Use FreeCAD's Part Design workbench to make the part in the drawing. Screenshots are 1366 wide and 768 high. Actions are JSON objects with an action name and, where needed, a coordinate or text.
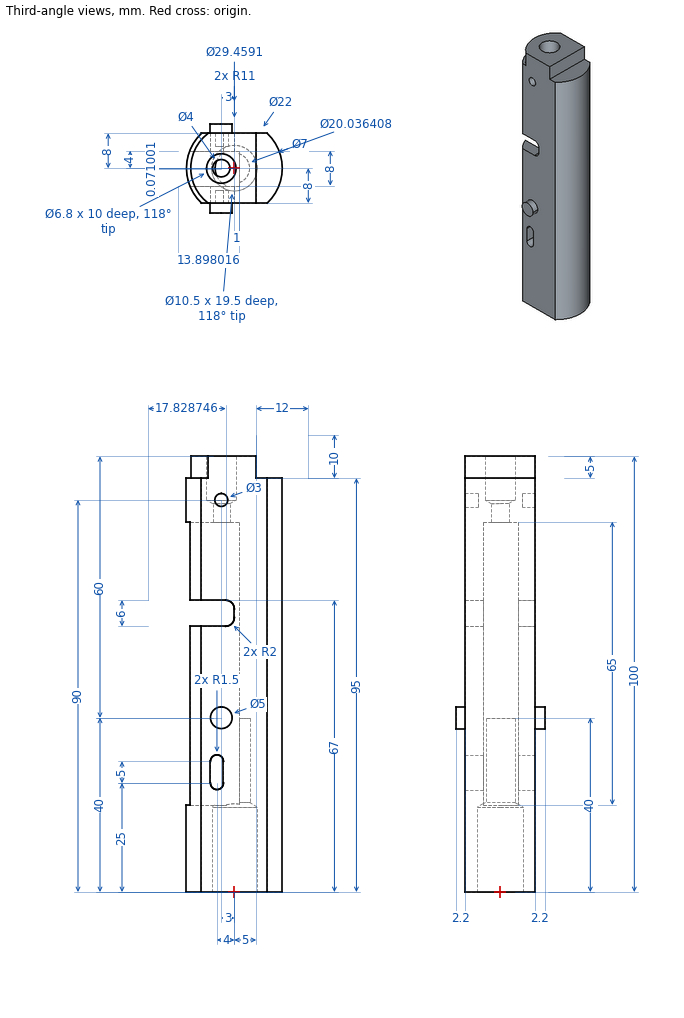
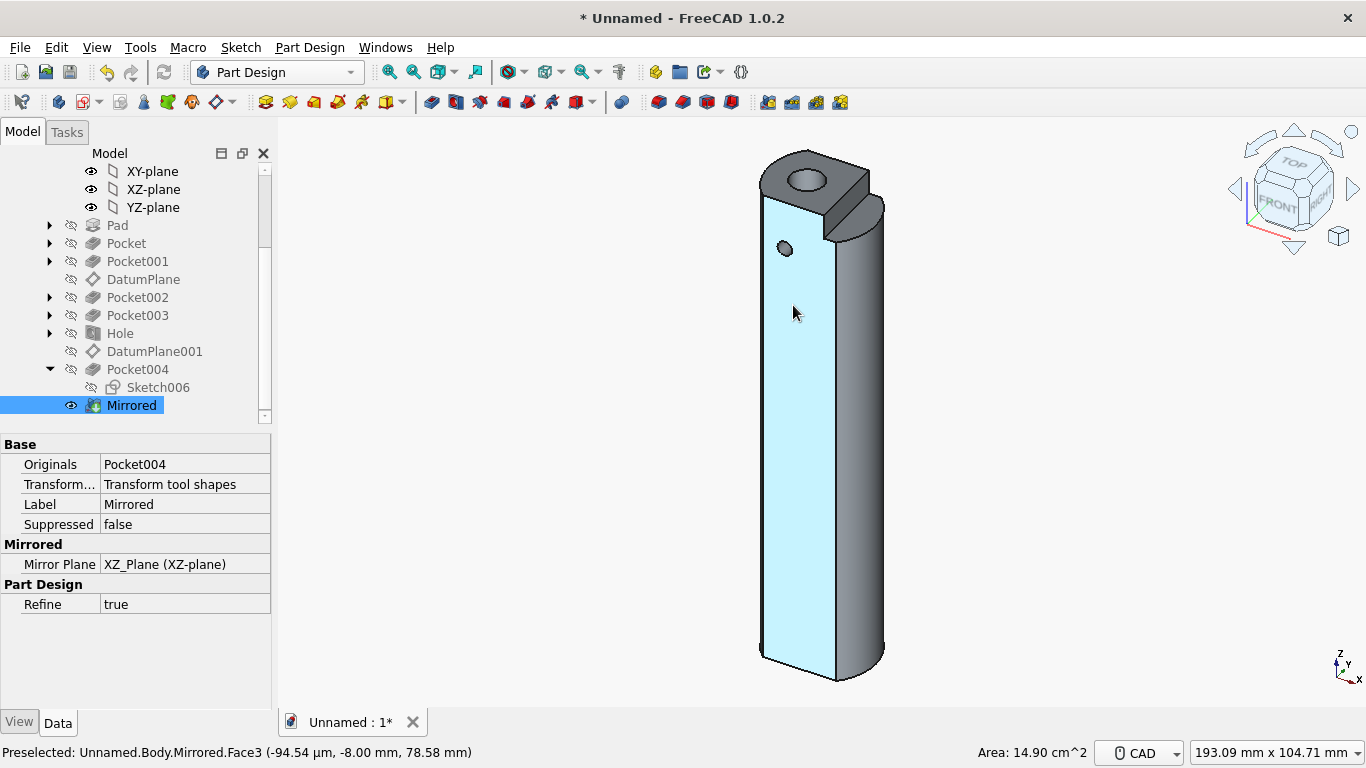
{"action": "left_click", "coordinate": [84, 102]}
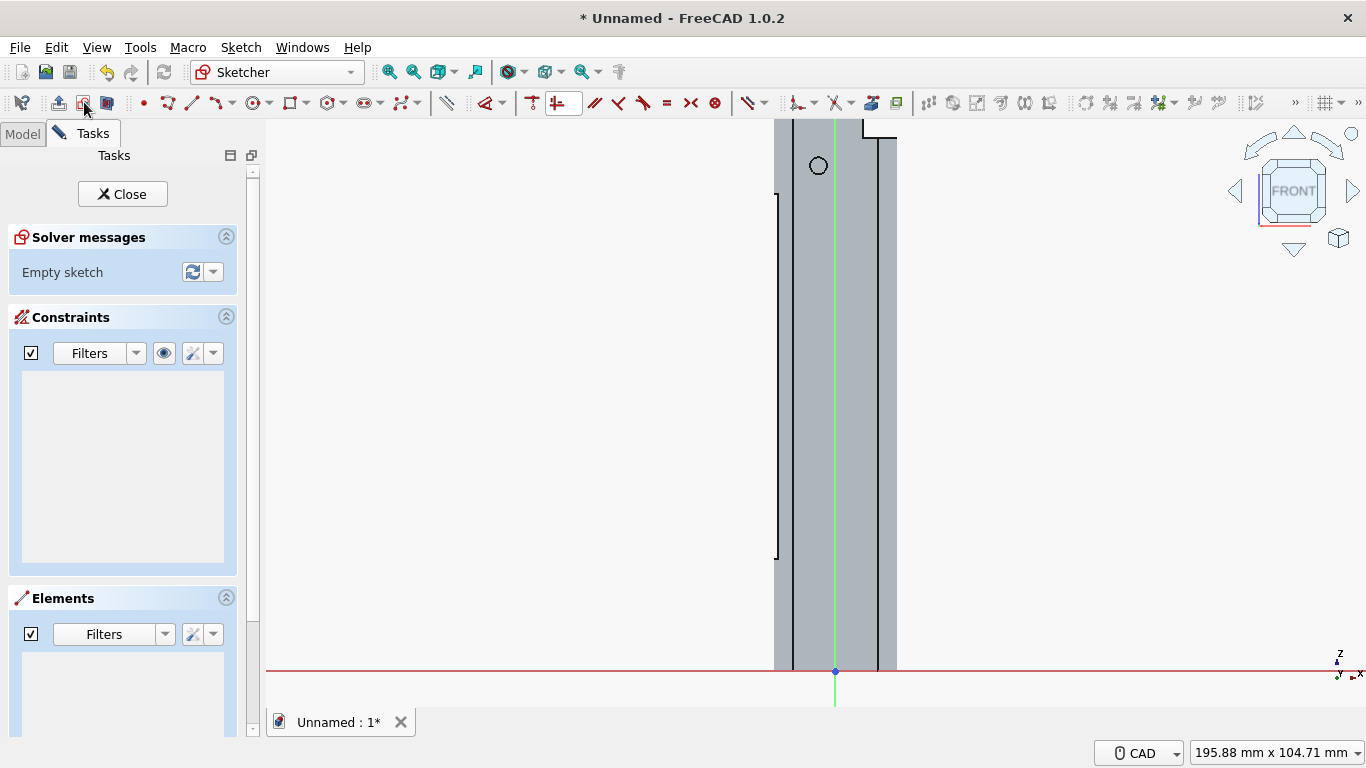
{"action": "scroll", "coordinate": [821, 530], "scroll_direction": "up", "scroll_amount": 11}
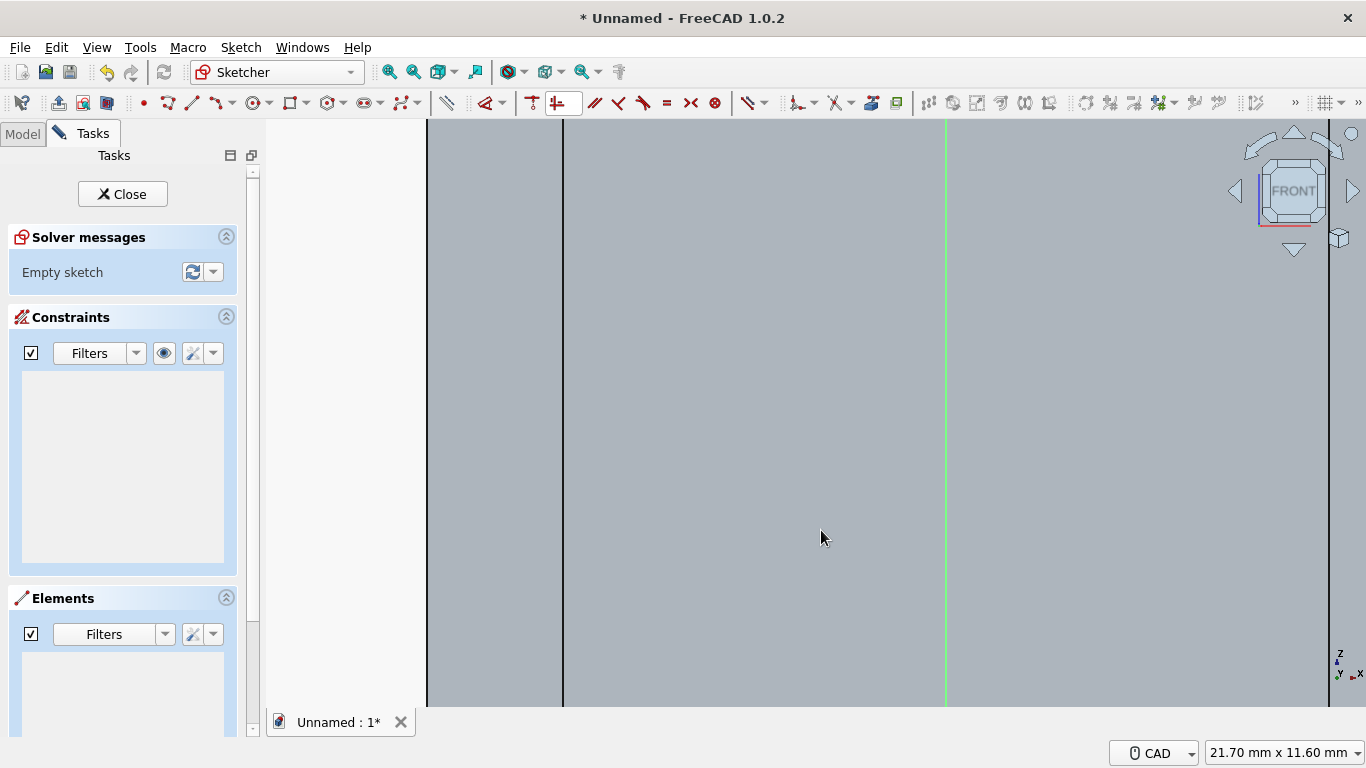
{"action": "key", "text": "g s"}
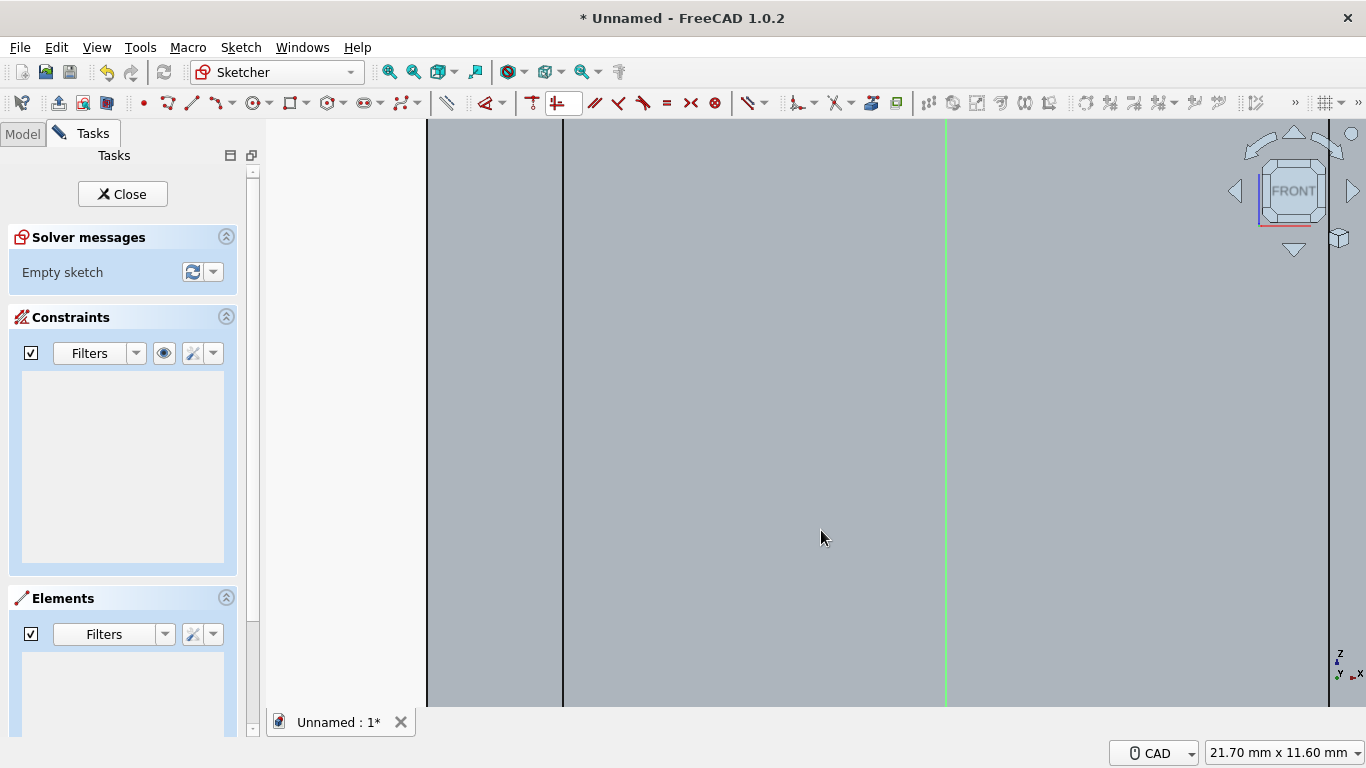
{"action": "left_click", "coordinate": [743, 532]}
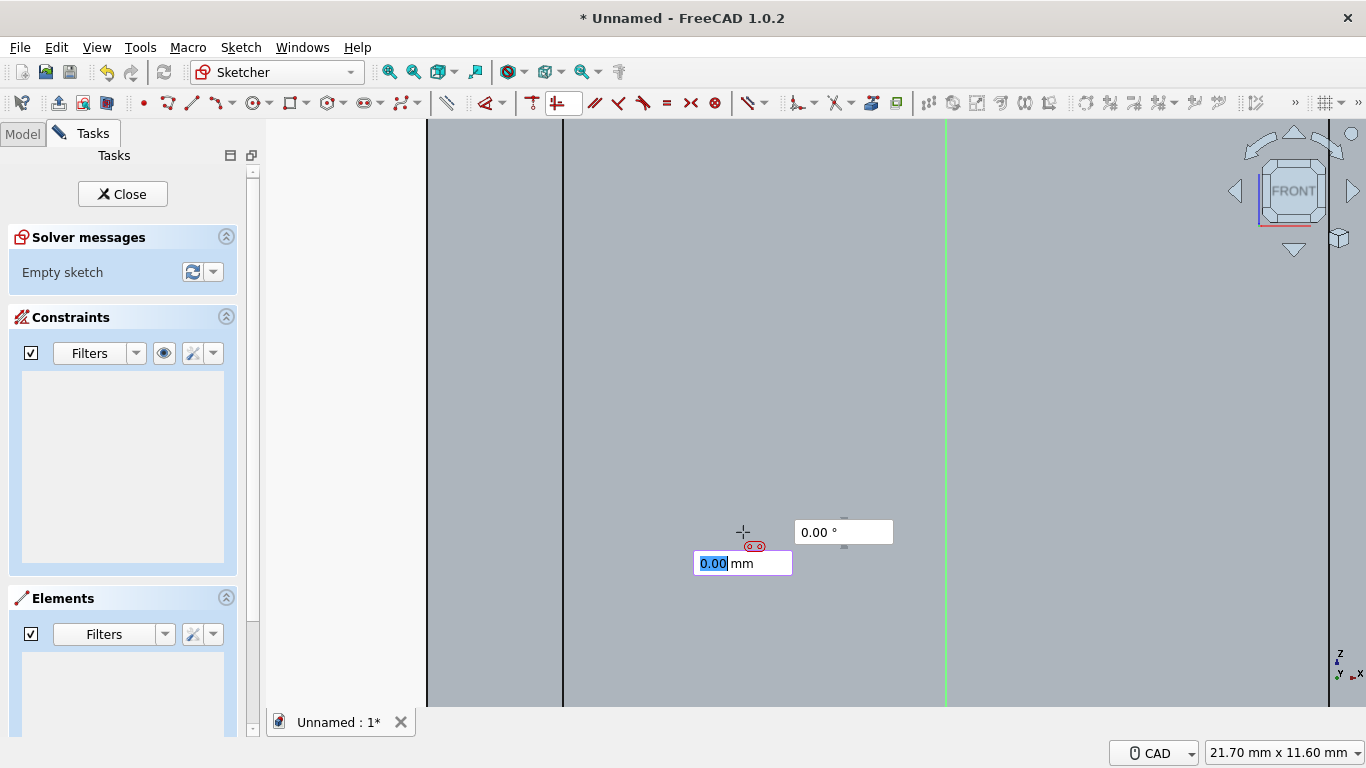
{"action": "left_click", "coordinate": [743, 278]}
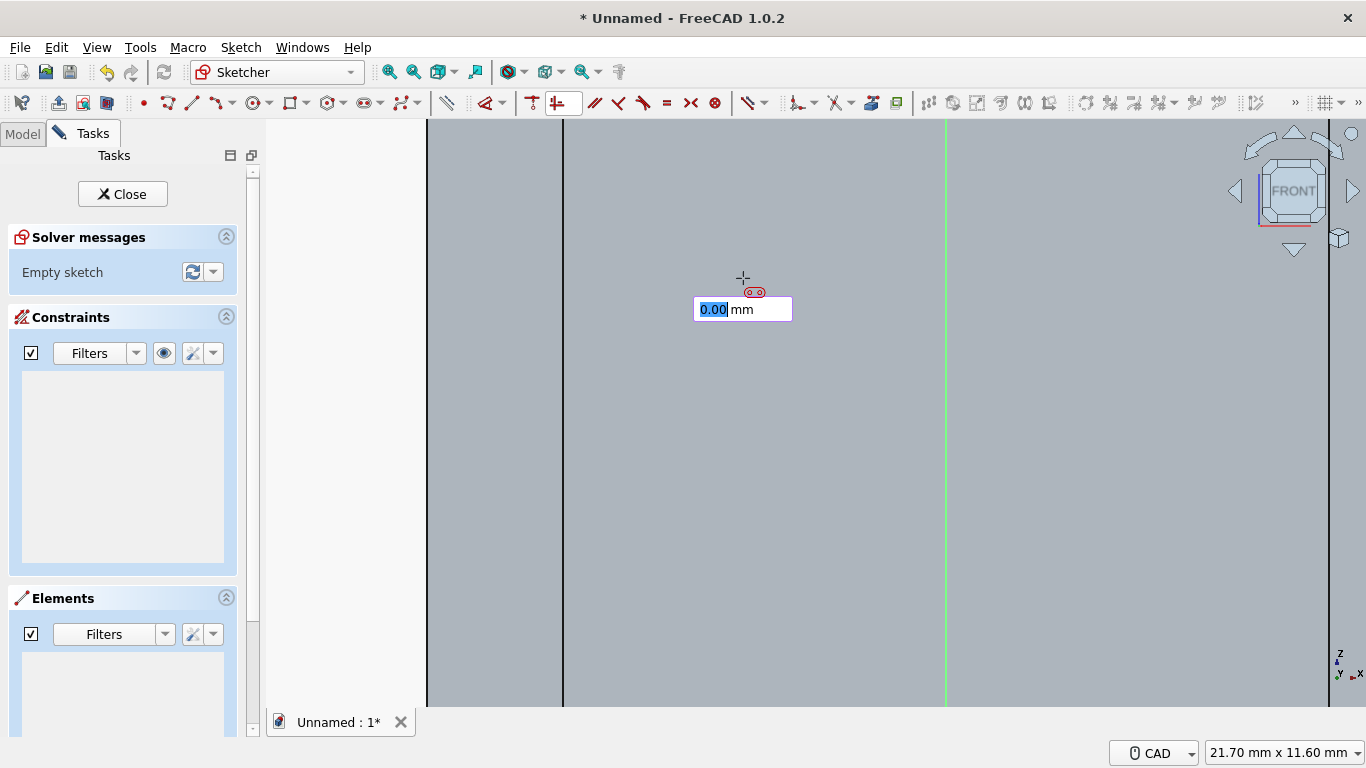
{"action": "left_click", "coordinate": [819, 405]}
{"action": "key", "text": "Escape"}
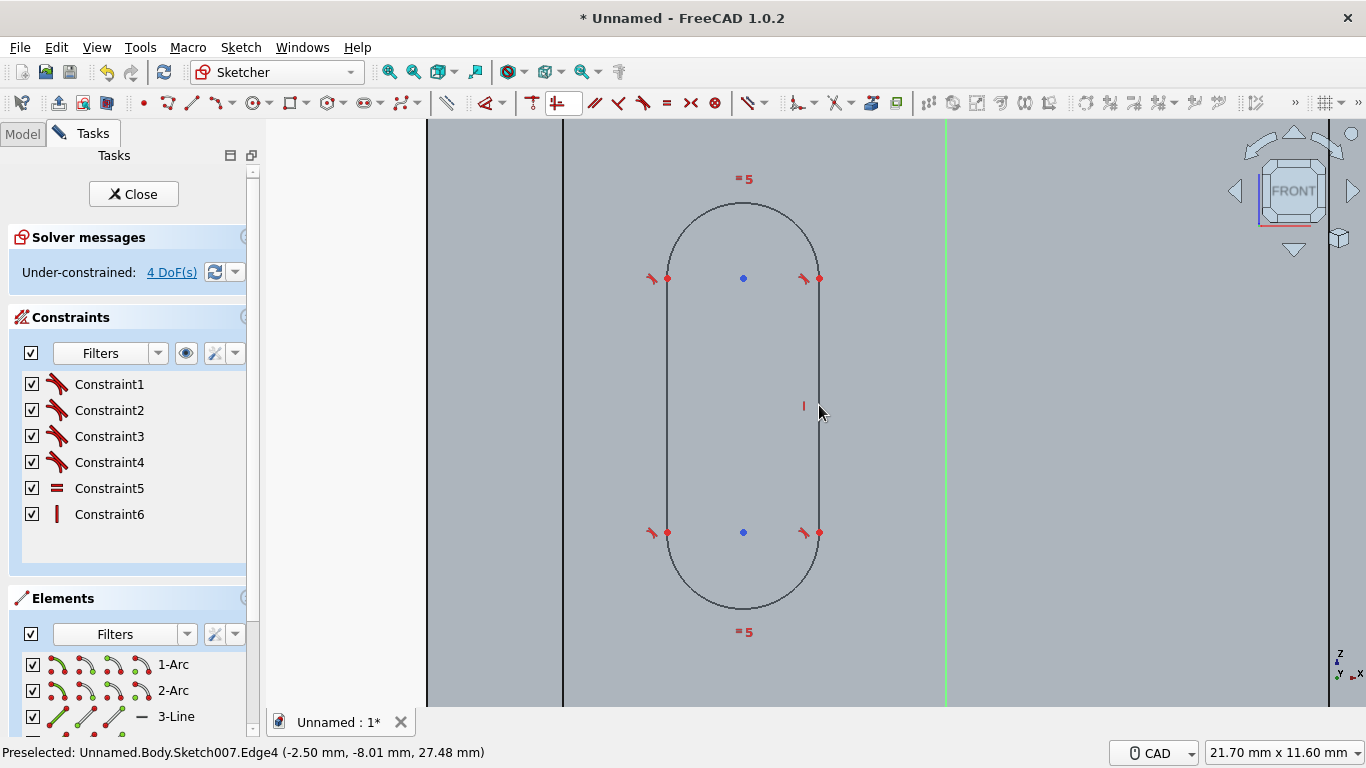
{"action": "left_click", "coordinate": [486, 104]}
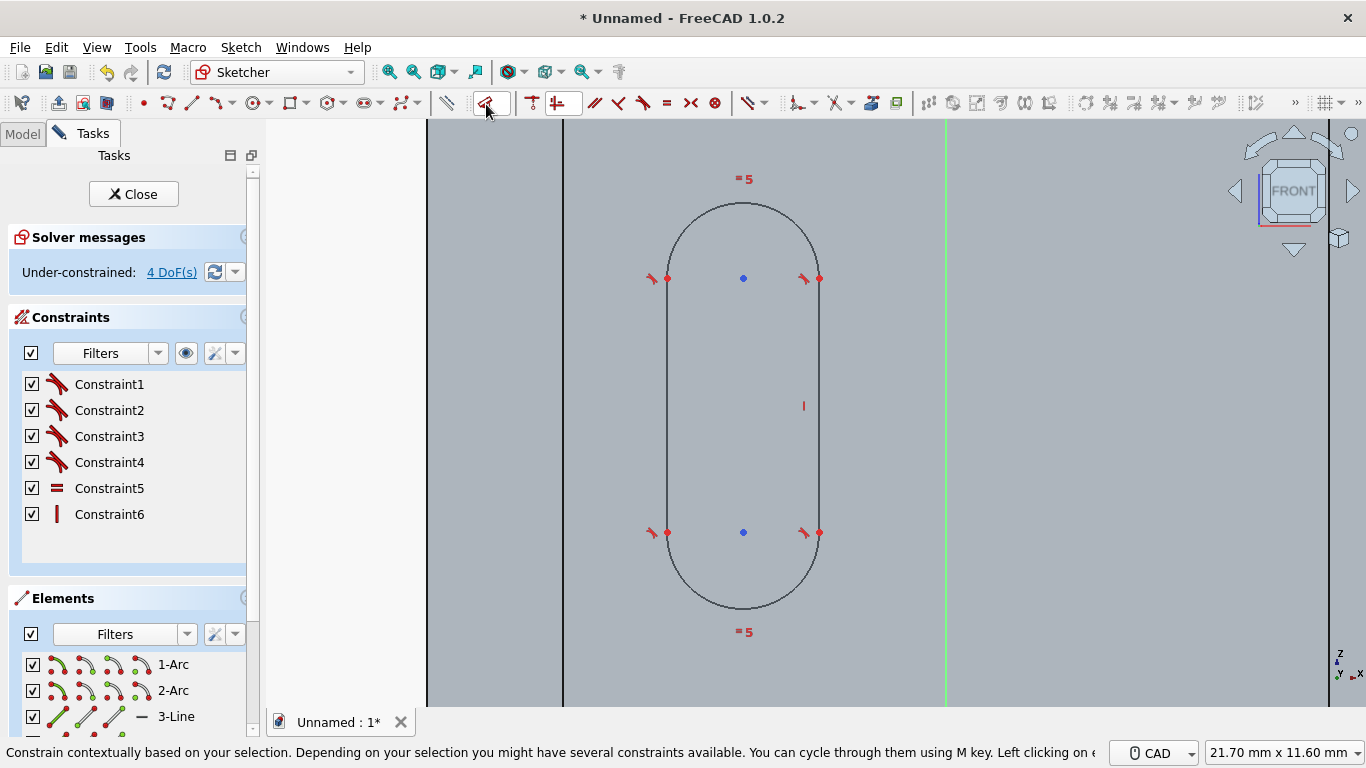
{"action": "left_click", "coordinate": [698, 594]}
{"action": "left_click", "coordinate": [679, 620]}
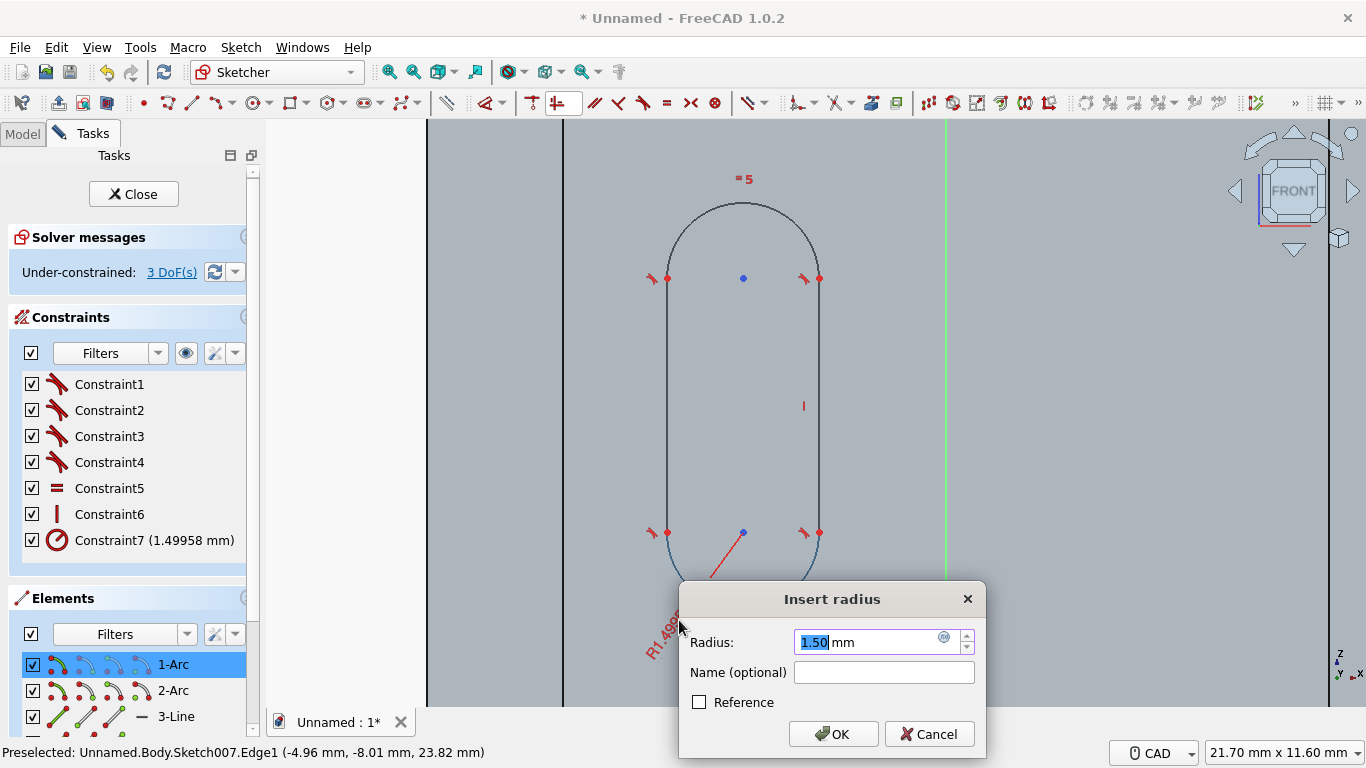
{"action": "type", "text": "1.5"}
{"action": "key", "text": "Return"}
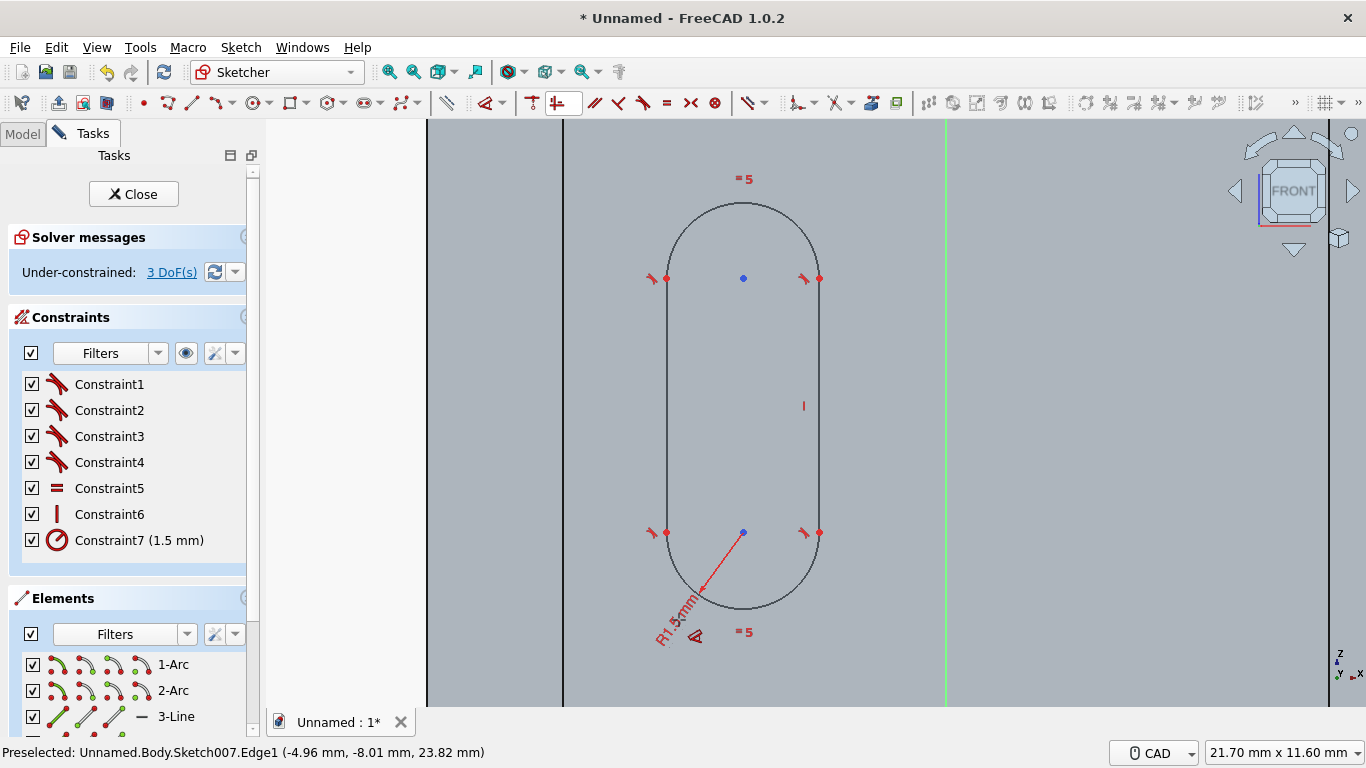
{"action": "left_click", "coordinate": [667, 457]}
{"action": "left_click", "coordinate": [633, 406]}